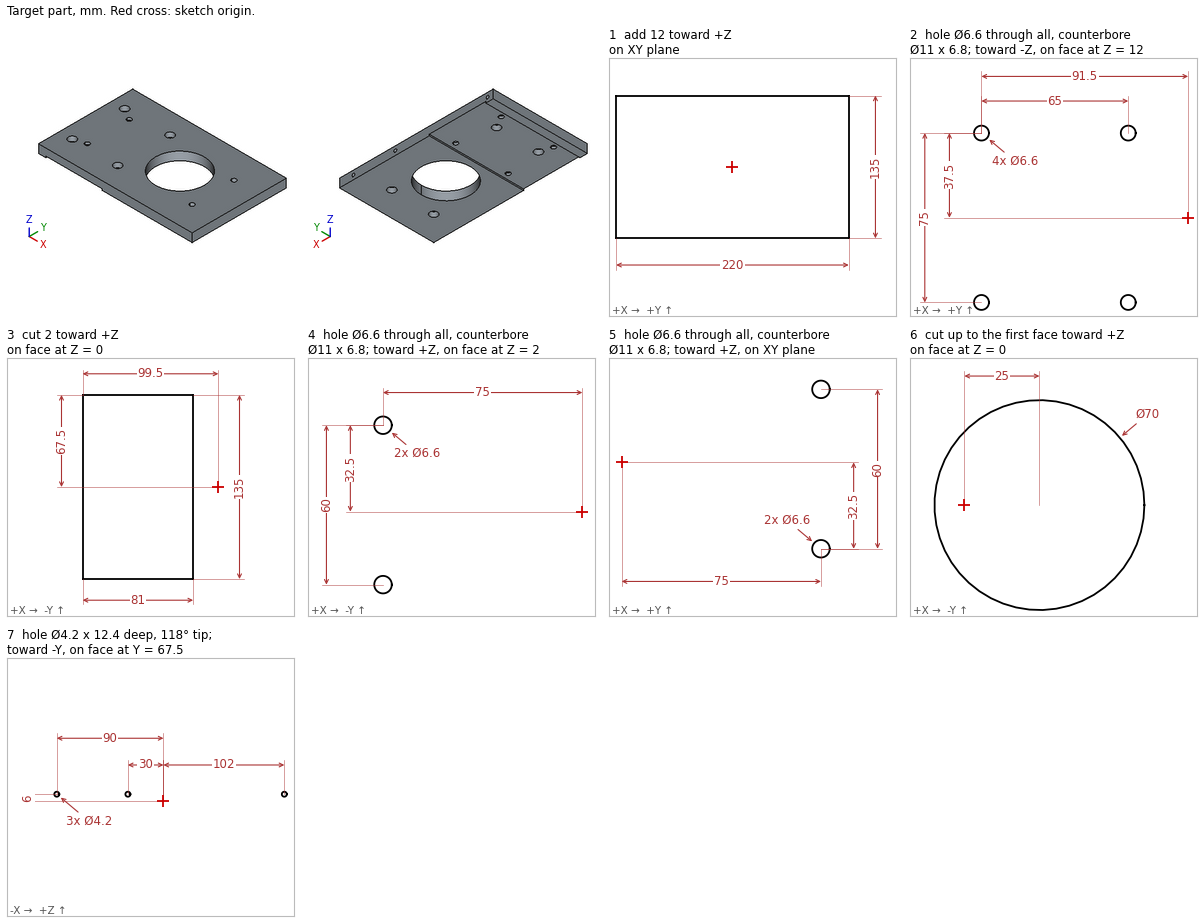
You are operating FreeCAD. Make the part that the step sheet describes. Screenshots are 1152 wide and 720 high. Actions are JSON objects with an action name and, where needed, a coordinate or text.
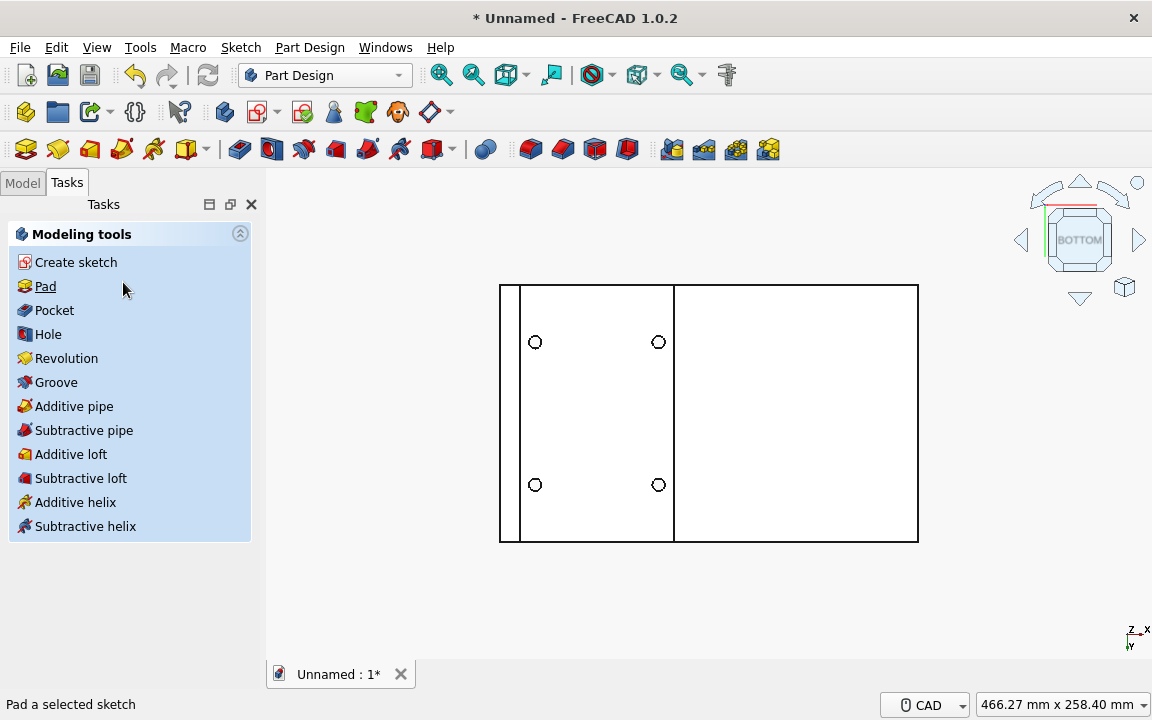
{"action": "left_click", "coordinate": [272, 150]}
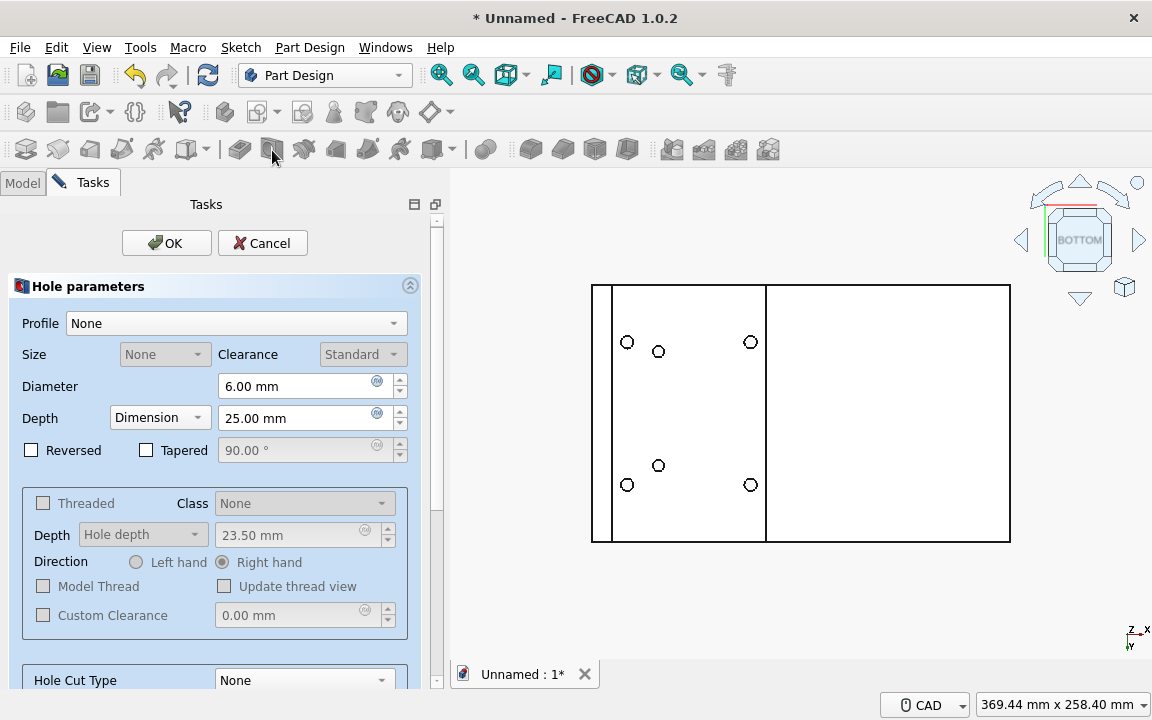
{"action": "triple_click", "coordinate": [305, 386]}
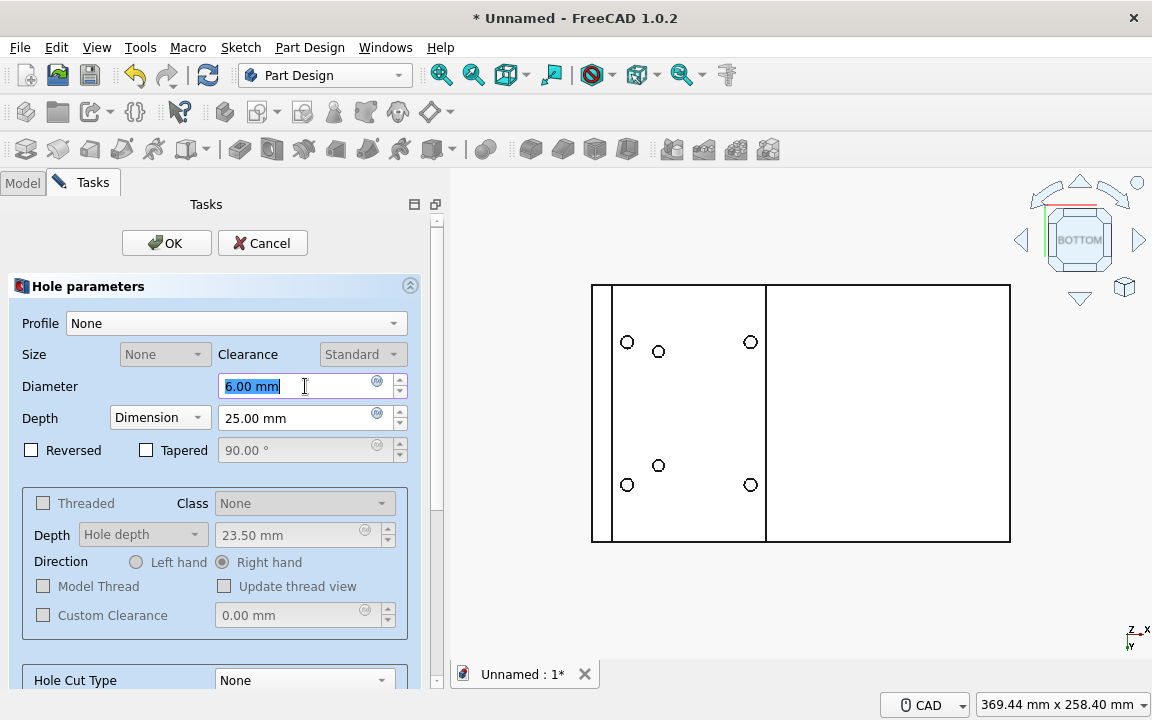
{"action": "type", "text": "6.6"}
{"action": "key", "text": "Tab"}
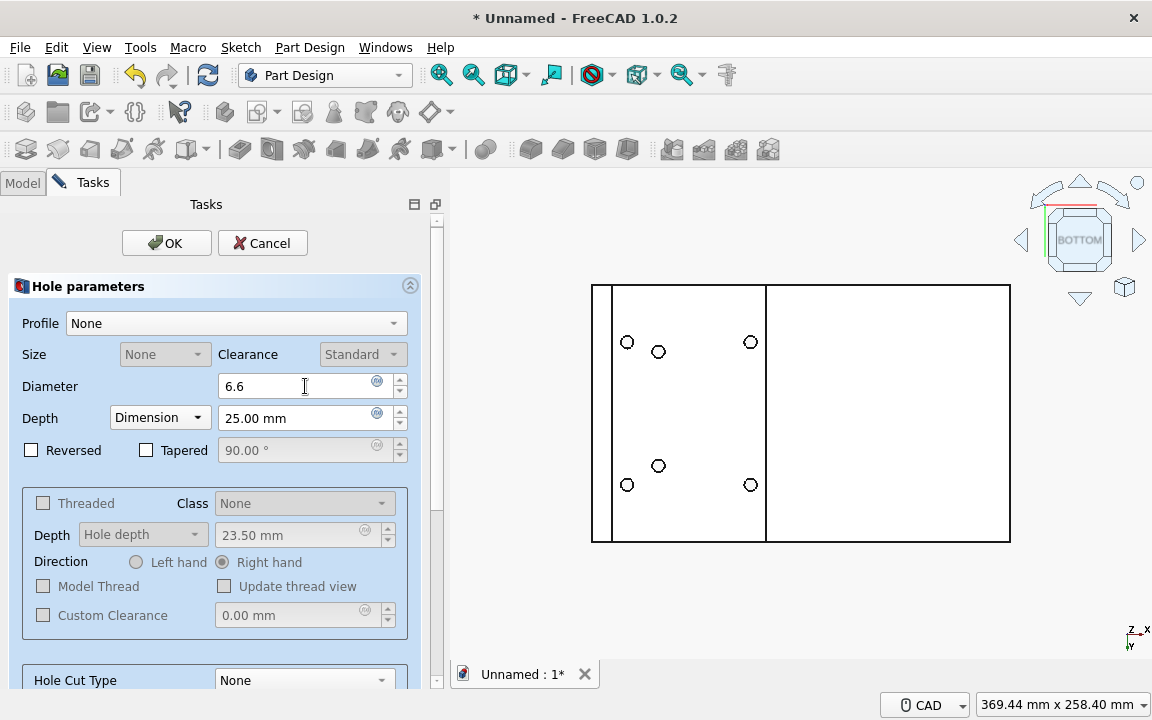
{"action": "left_click", "coordinate": [161, 418]}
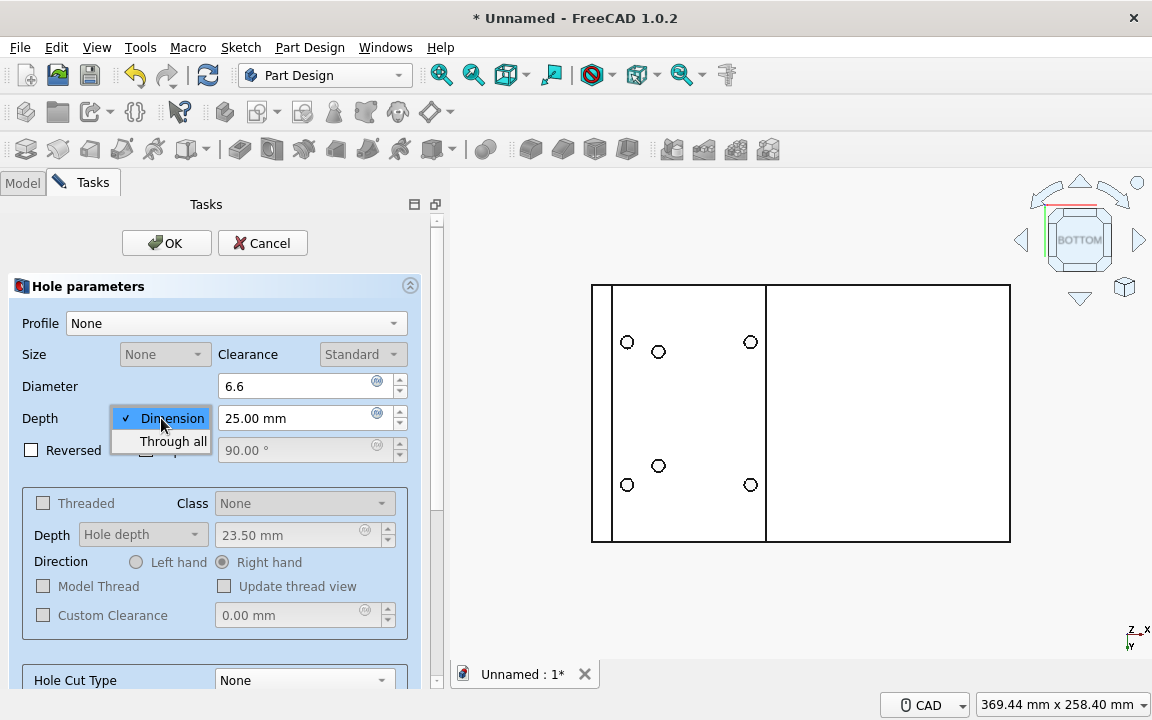
{"action": "left_click", "coordinate": [160, 442]}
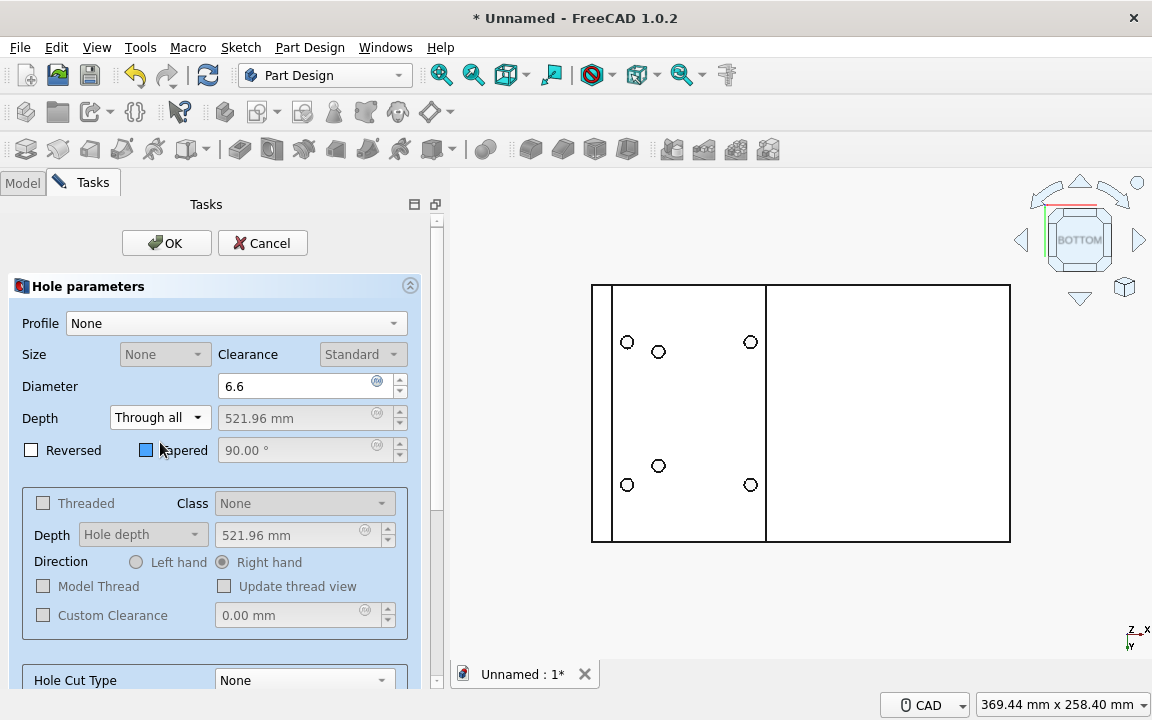
{"action": "scroll", "coordinate": [437, 451], "scroll_direction": "down", "scroll_amount": 2}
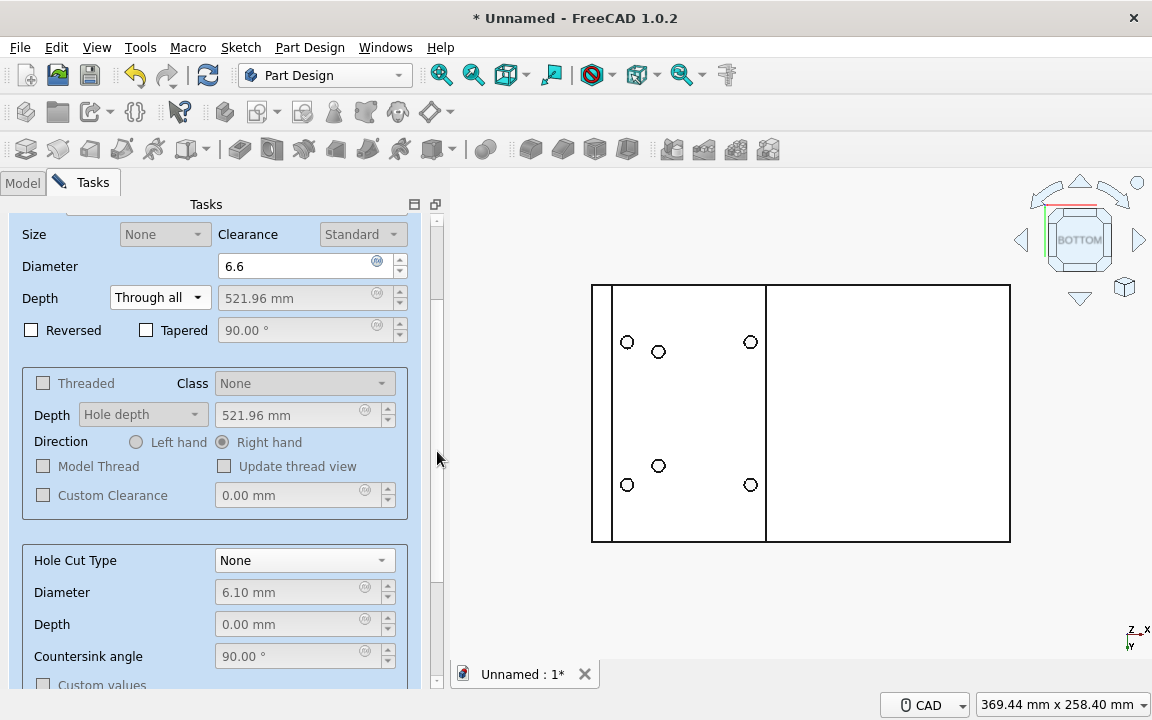
{"action": "left_click", "coordinate": [306, 560]}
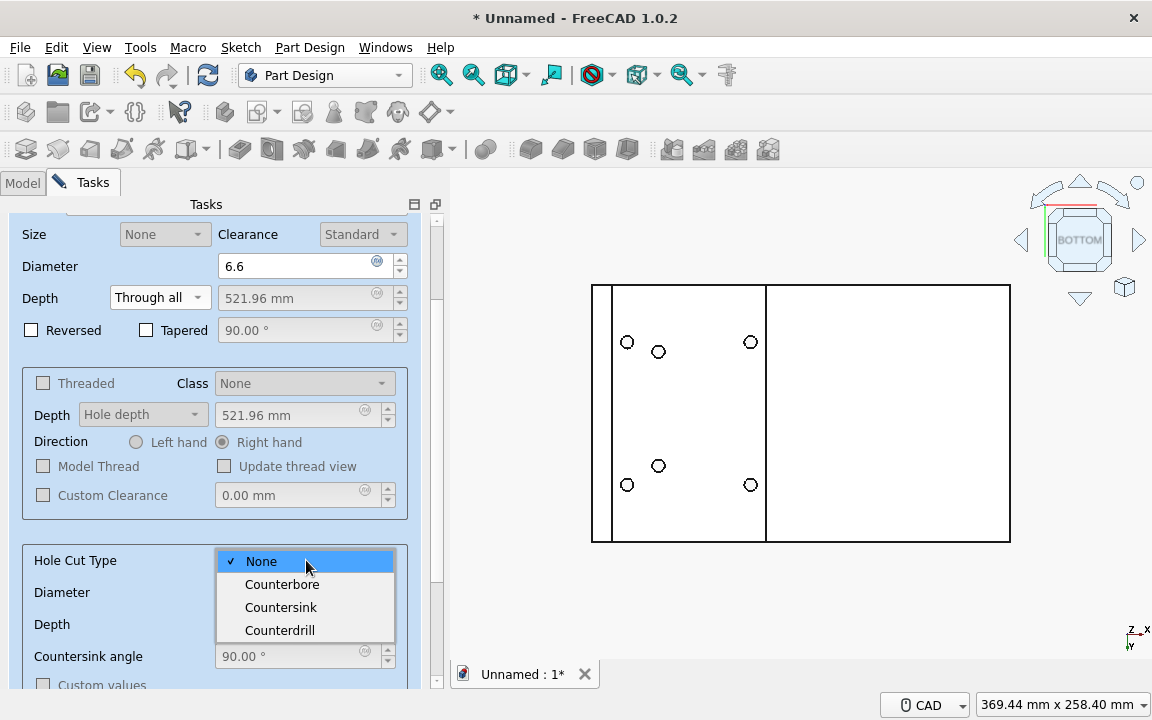
{"action": "left_click", "coordinate": [304, 584]}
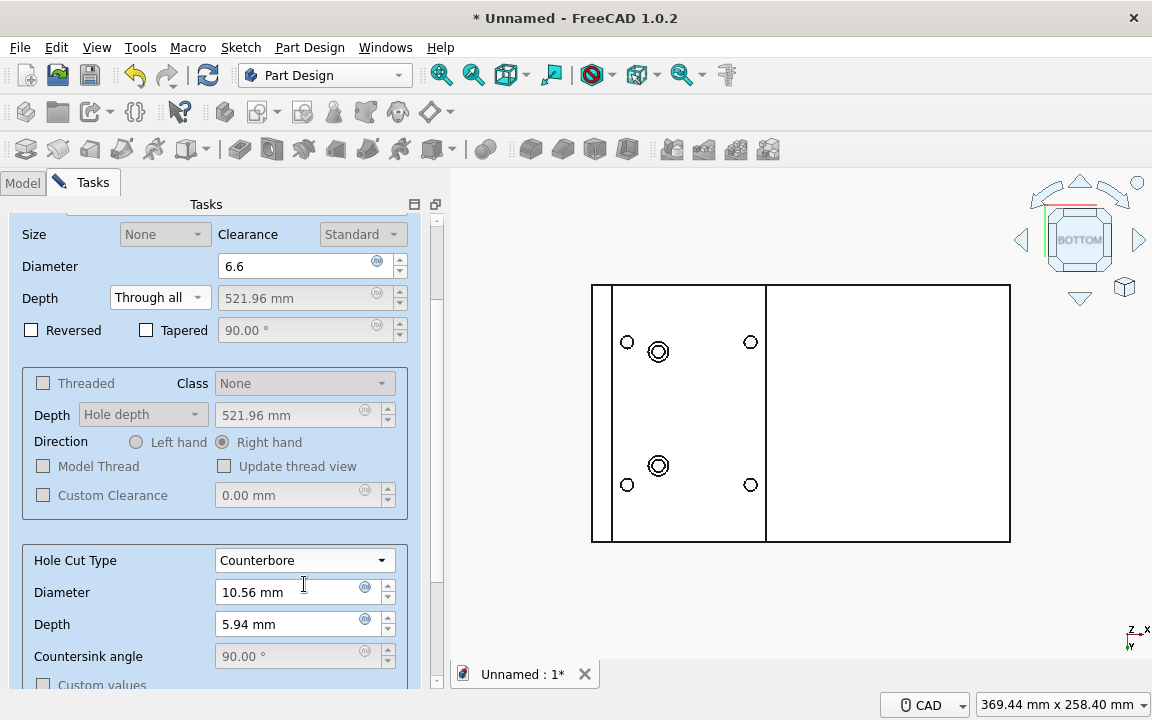
{"action": "triple_click", "coordinate": [298, 592]}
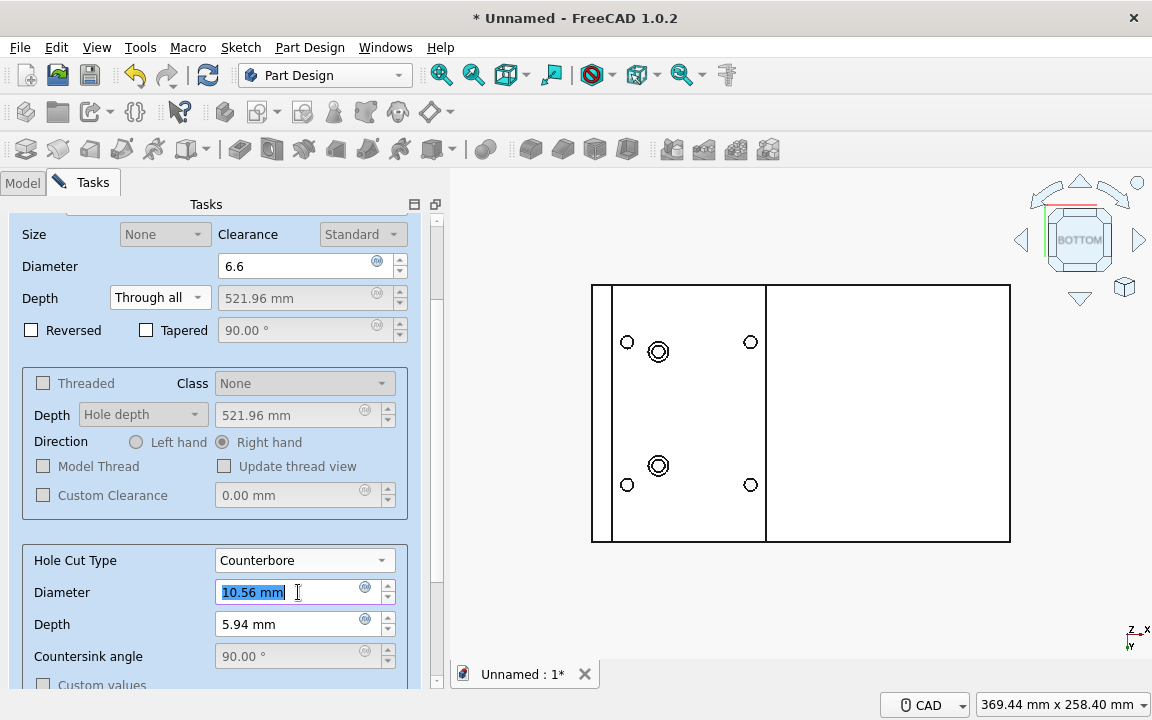
{"action": "type", "text": "11"}
{"action": "key", "text": "Tab"}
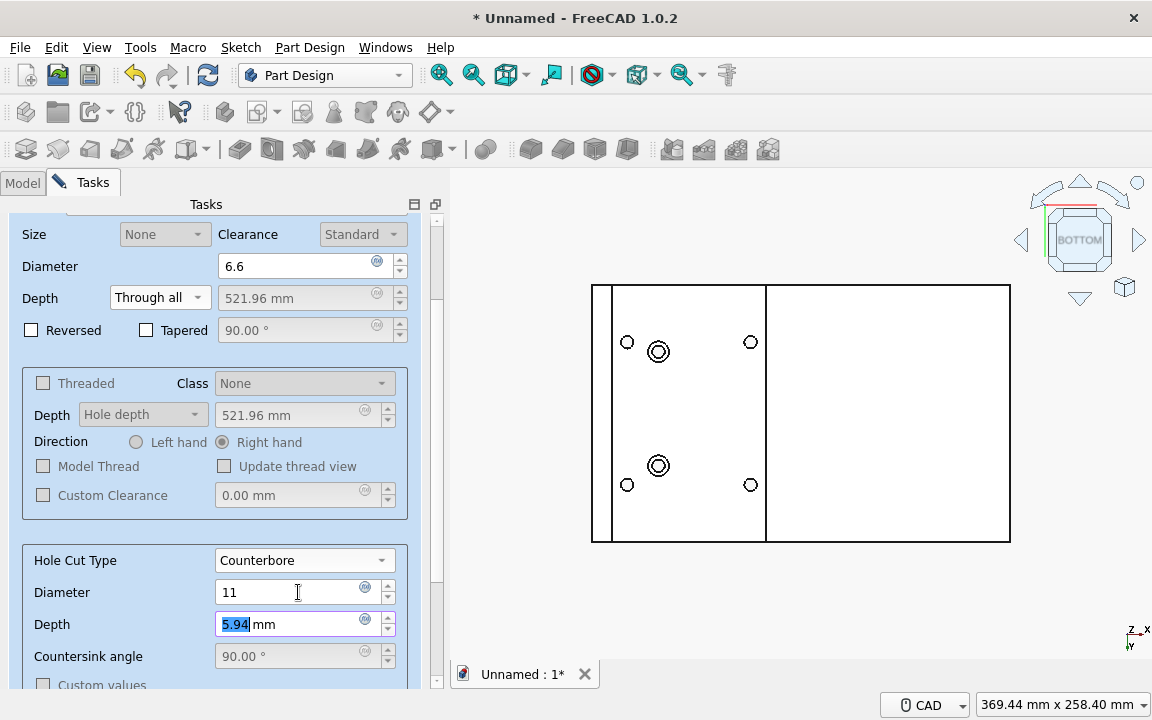
{"action": "type", "text": "6.8"}
{"action": "key", "text": "Tab"}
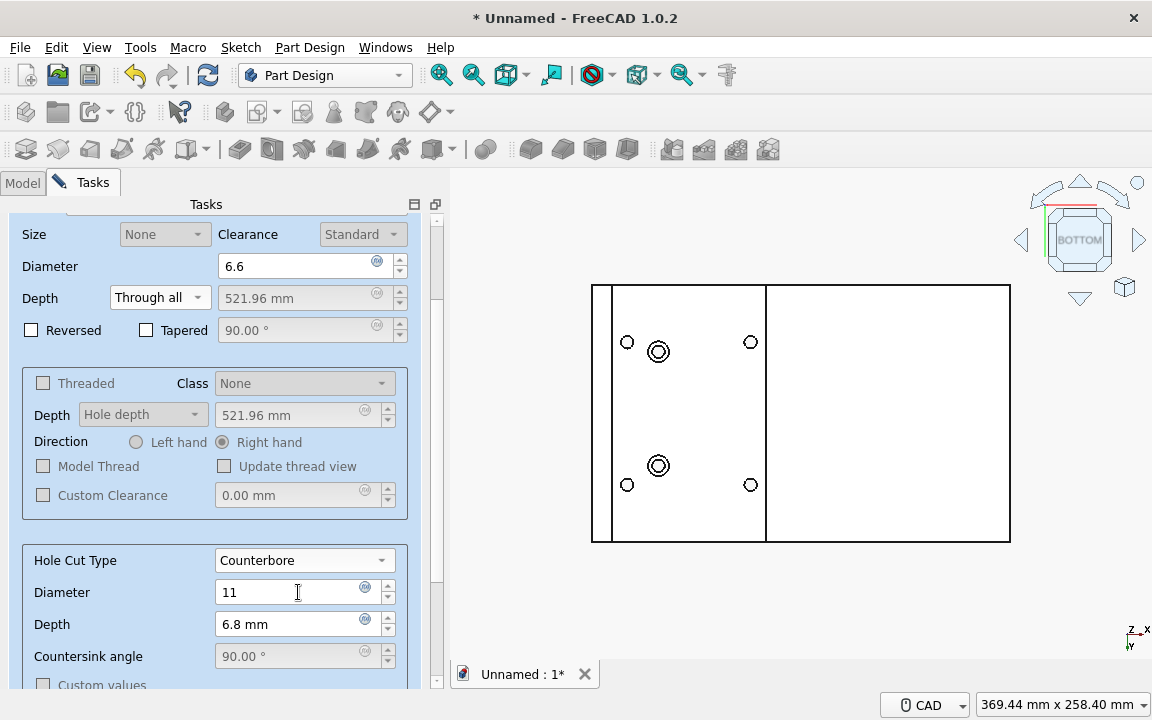
{"action": "scroll", "coordinate": [437, 451], "scroll_direction": "up", "scroll_amount": 3}